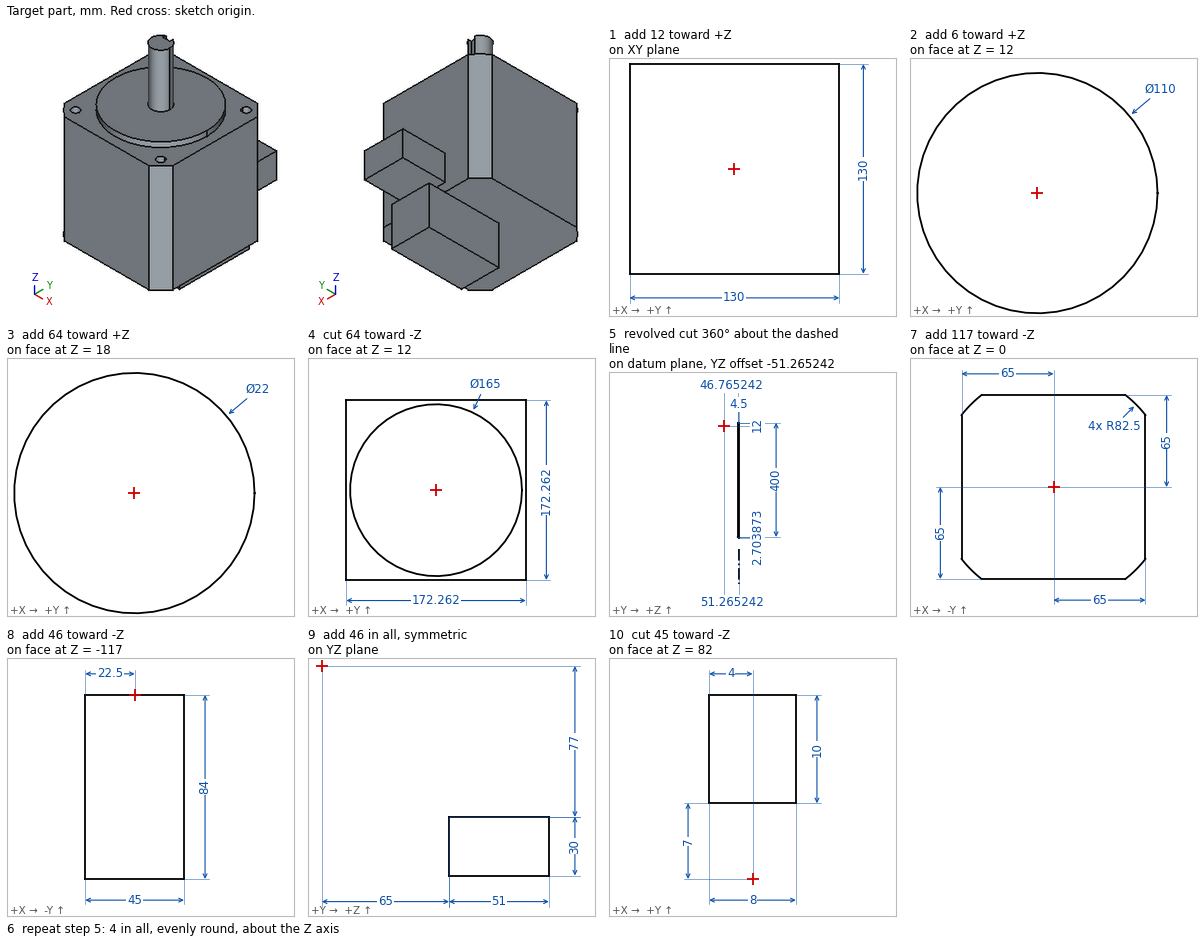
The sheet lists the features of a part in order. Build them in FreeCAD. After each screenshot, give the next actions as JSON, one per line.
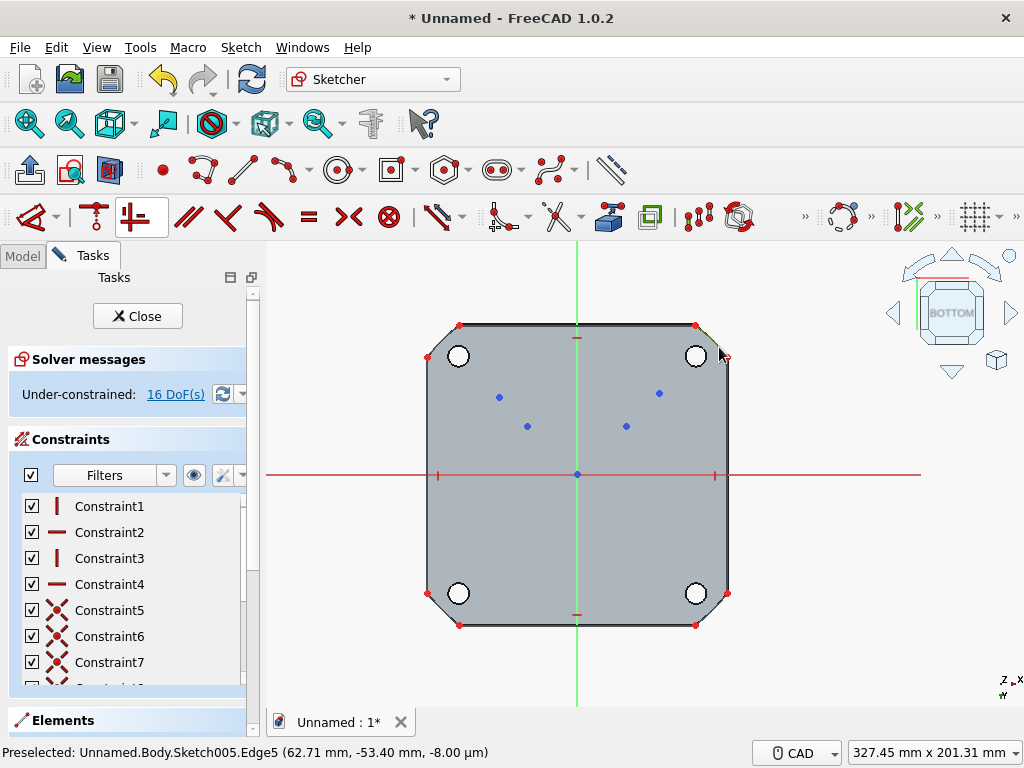
{"action": "left_click", "coordinate": [449, 334]}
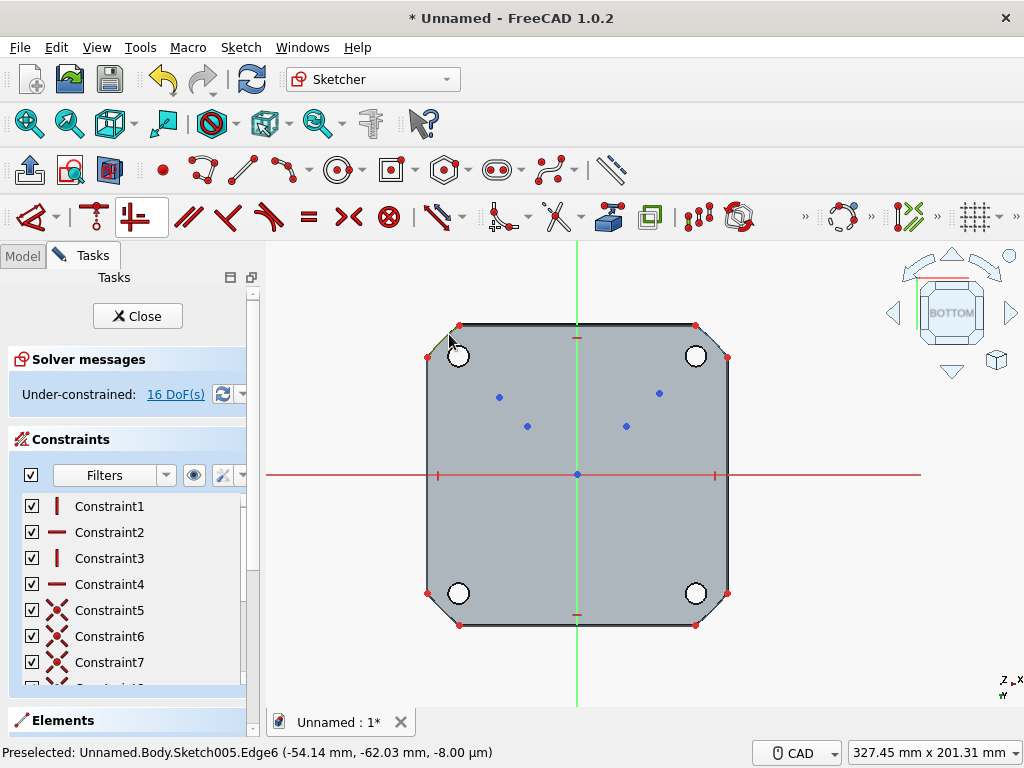
{"action": "left_click", "coordinate": [94, 218]}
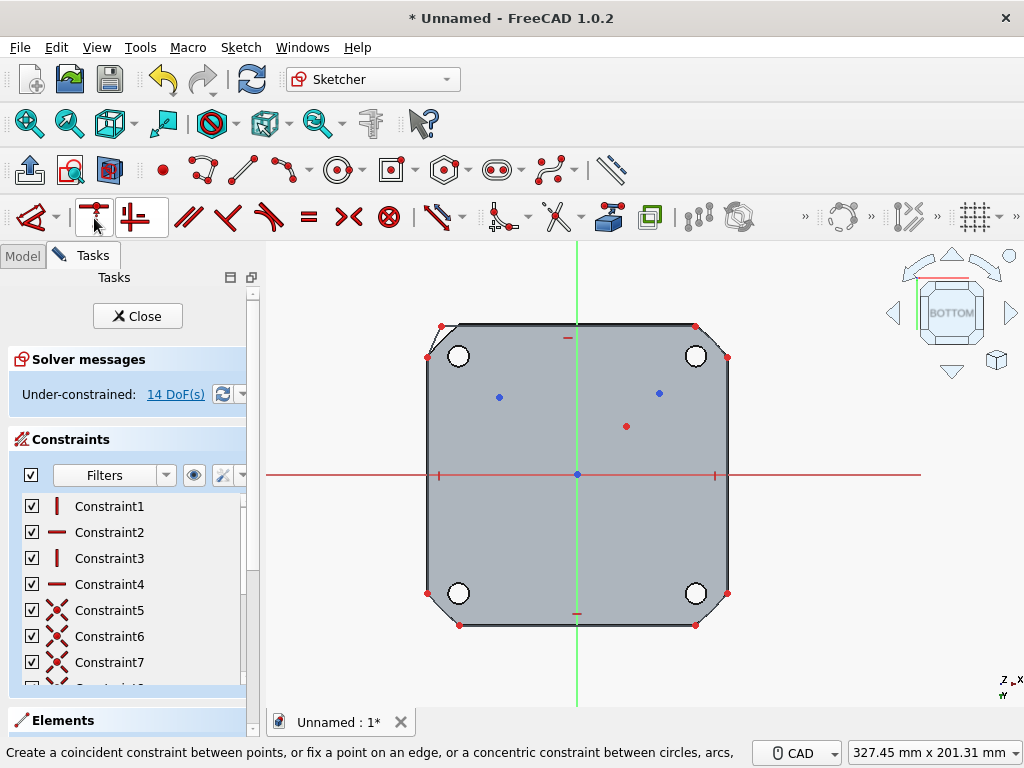
{"action": "left_click", "coordinate": [719, 347]}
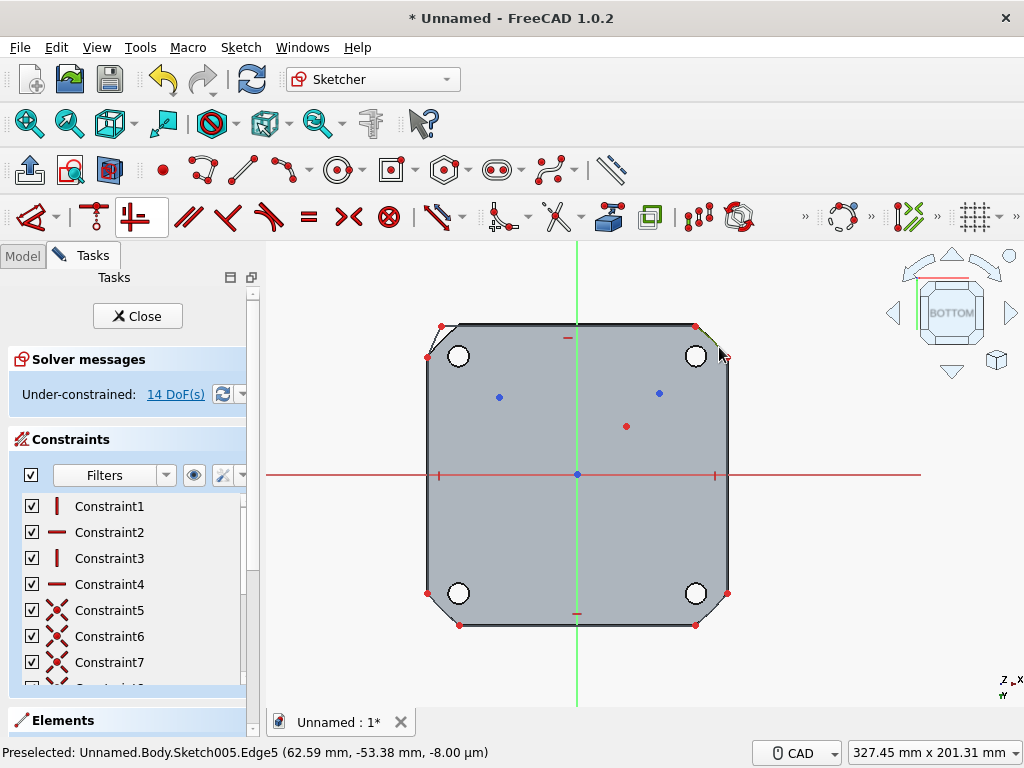
{"action": "left_click", "coordinate": [437, 604]}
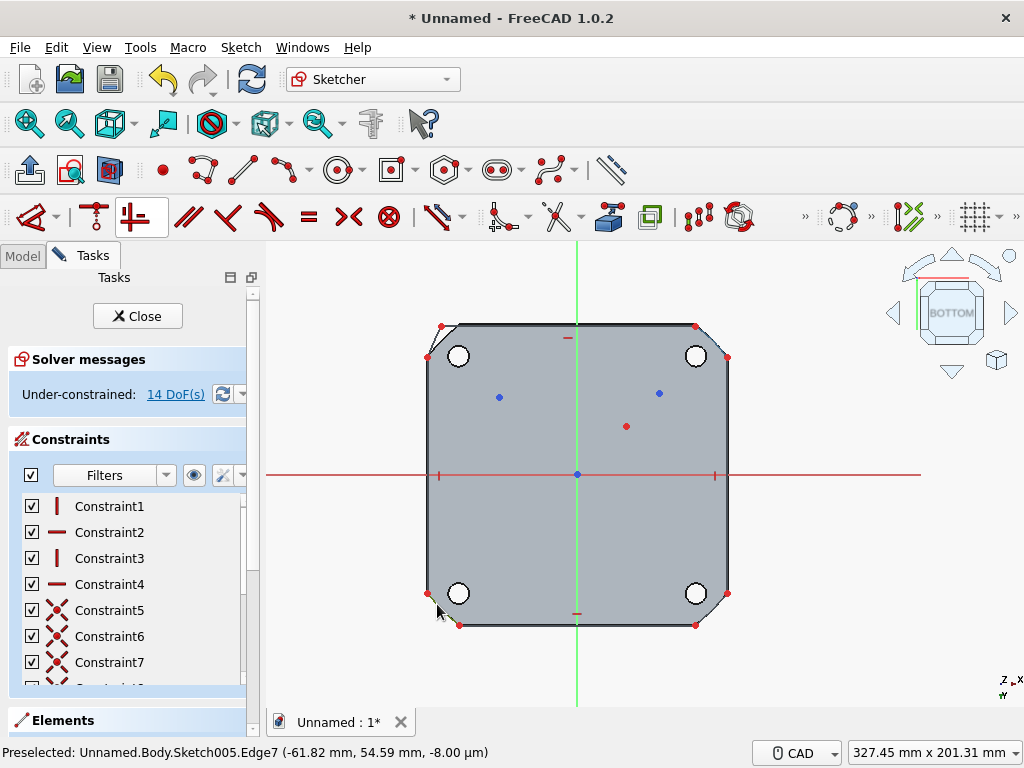
{"action": "left_click", "coordinate": [94, 218]}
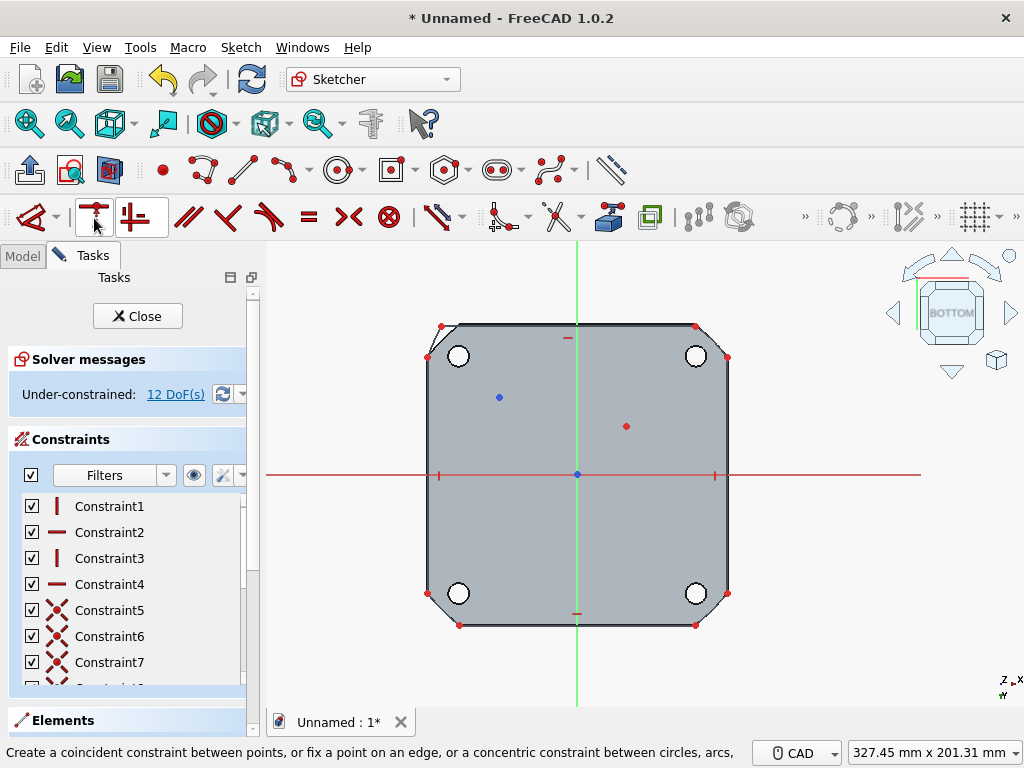
{"action": "left_click", "coordinate": [719, 347]}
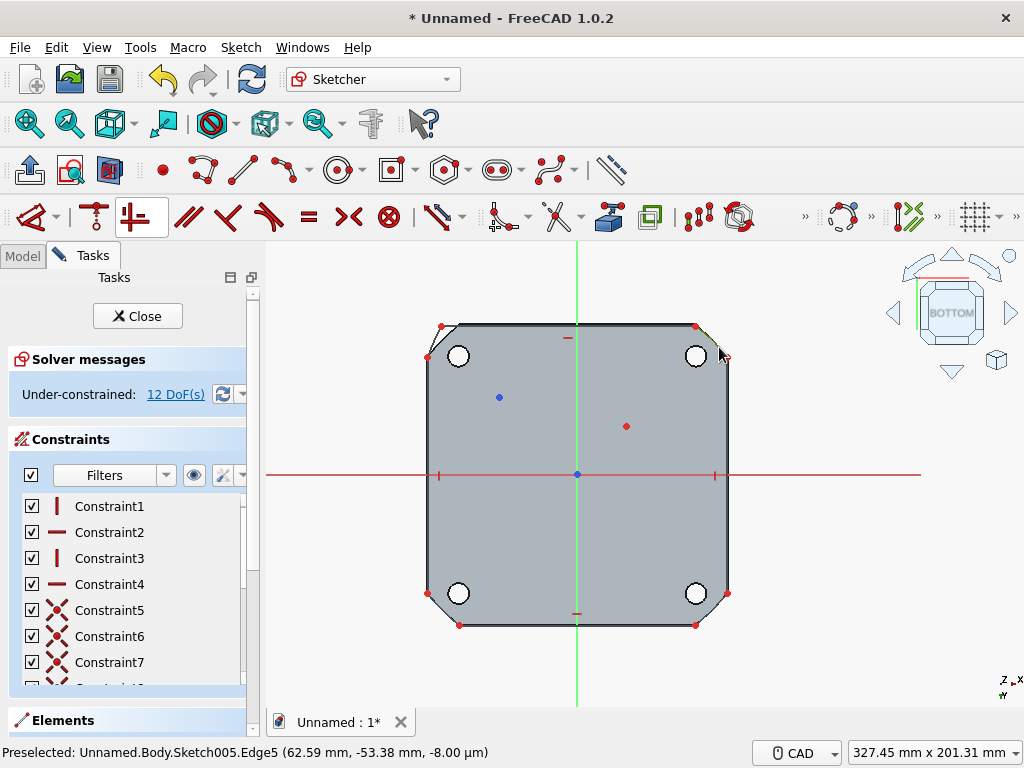
{"action": "left_click", "coordinate": [705, 617]}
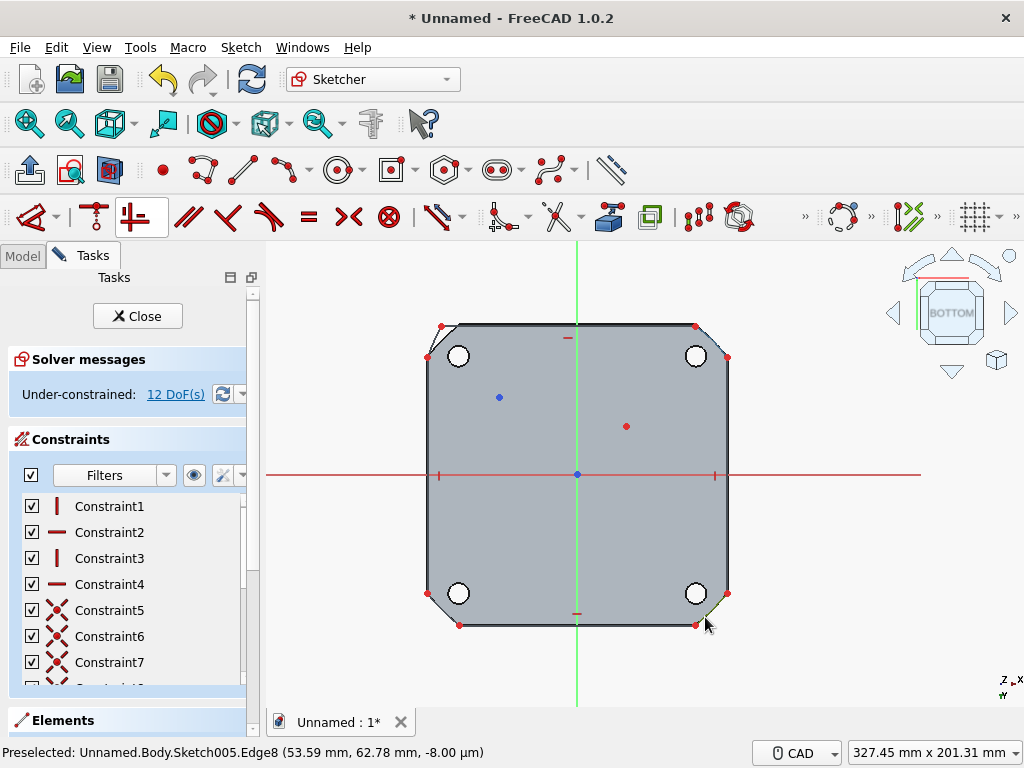
{"action": "left_click", "coordinate": [94, 218]}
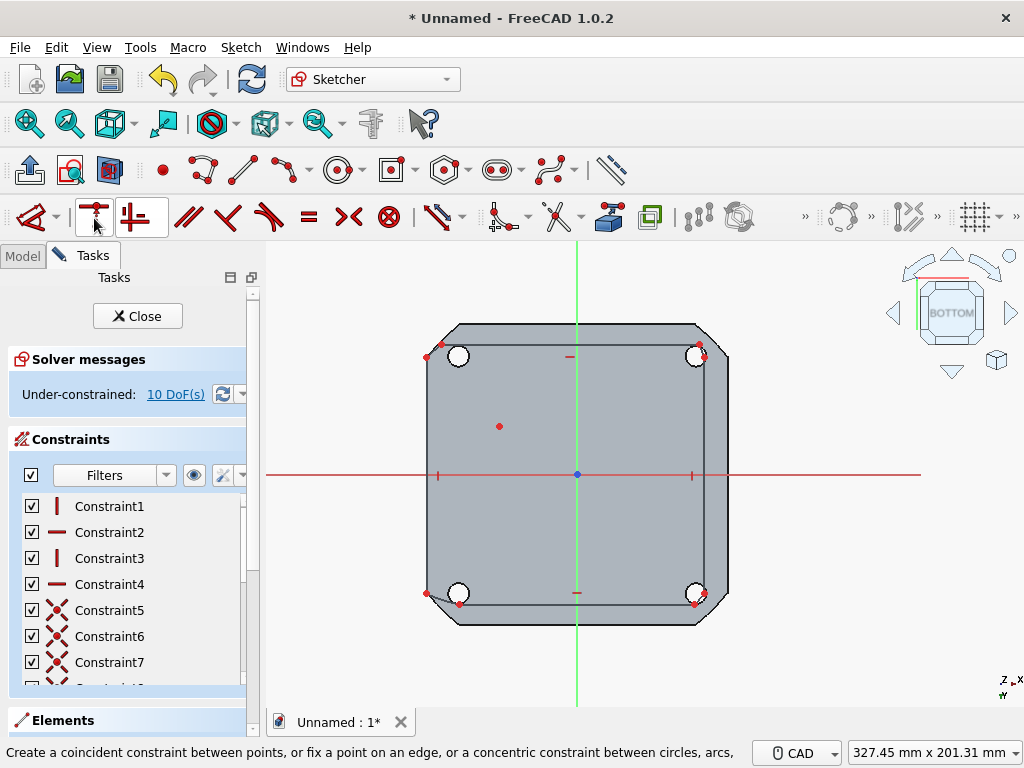
{"action": "left_click_drag", "start_coordinate": [489, 416], "coordinate": [587, 485]}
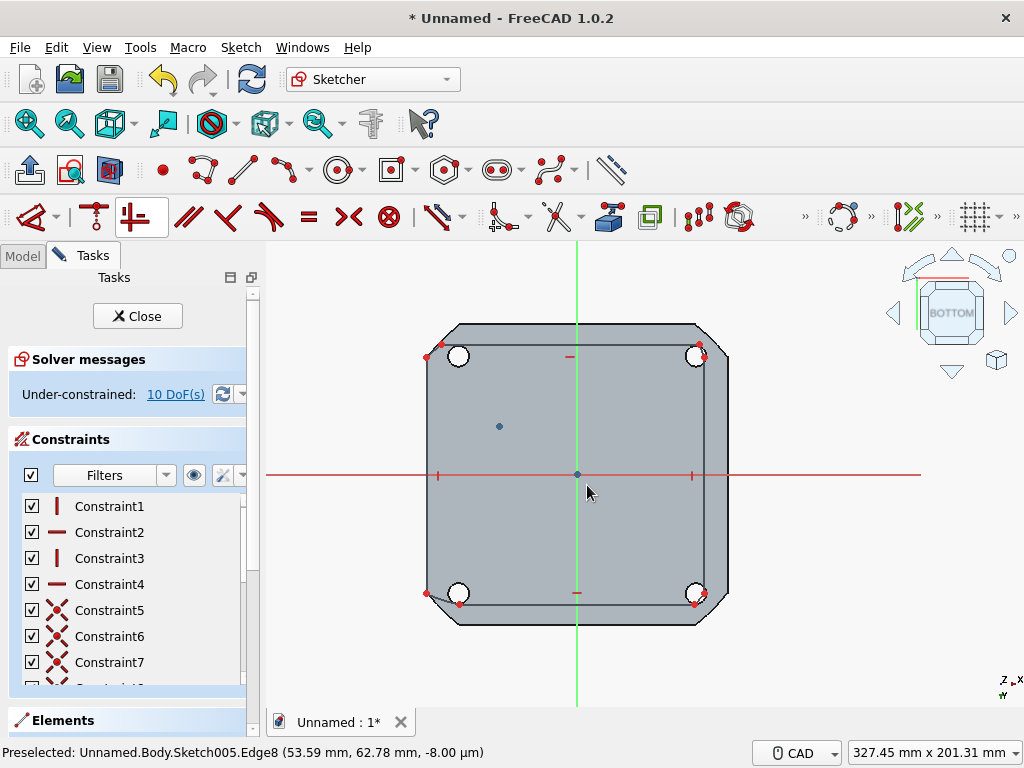
{"action": "key", "text": "c"}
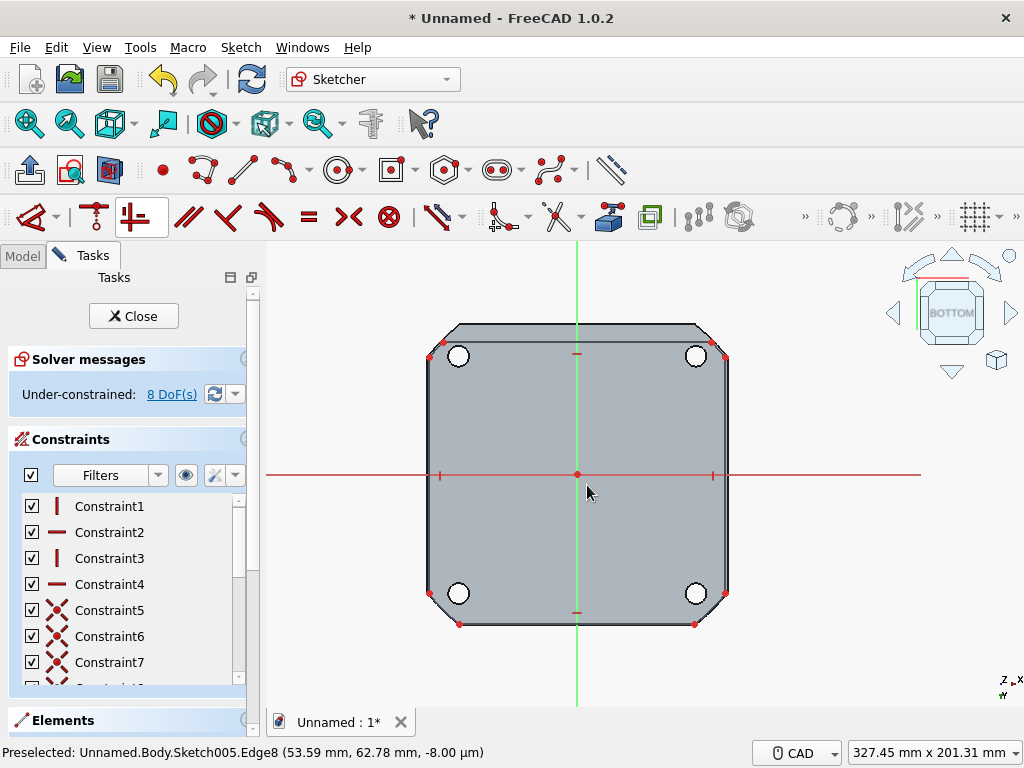
{"action": "scroll", "coordinate": [718, 350], "scroll_direction": "up", "scroll_amount": 2}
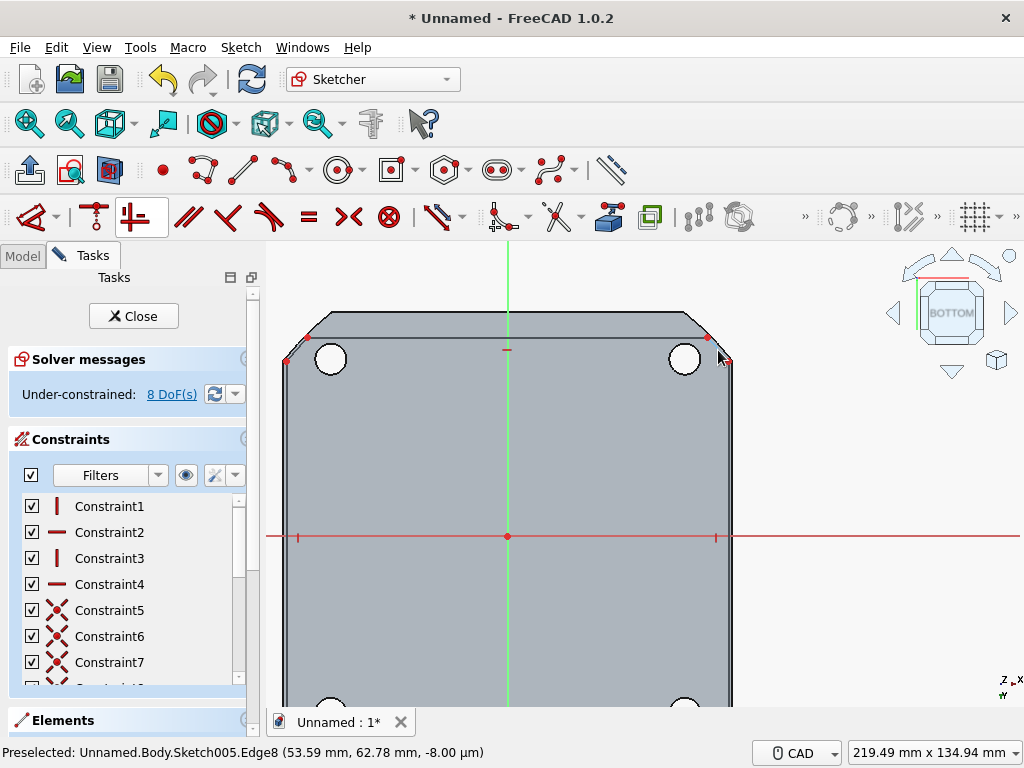
{"action": "left_click", "coordinate": [718, 350]}